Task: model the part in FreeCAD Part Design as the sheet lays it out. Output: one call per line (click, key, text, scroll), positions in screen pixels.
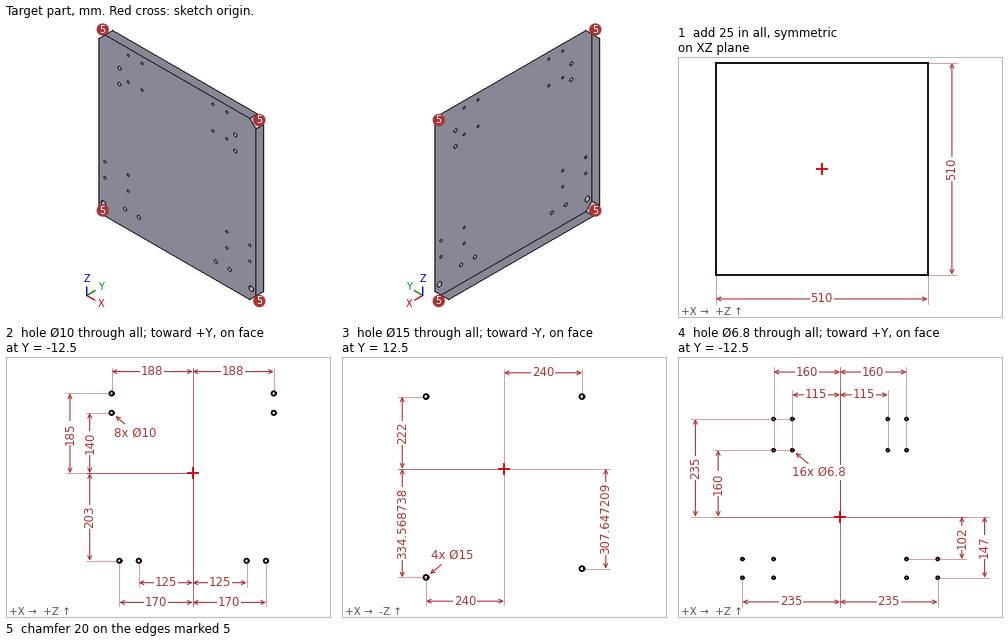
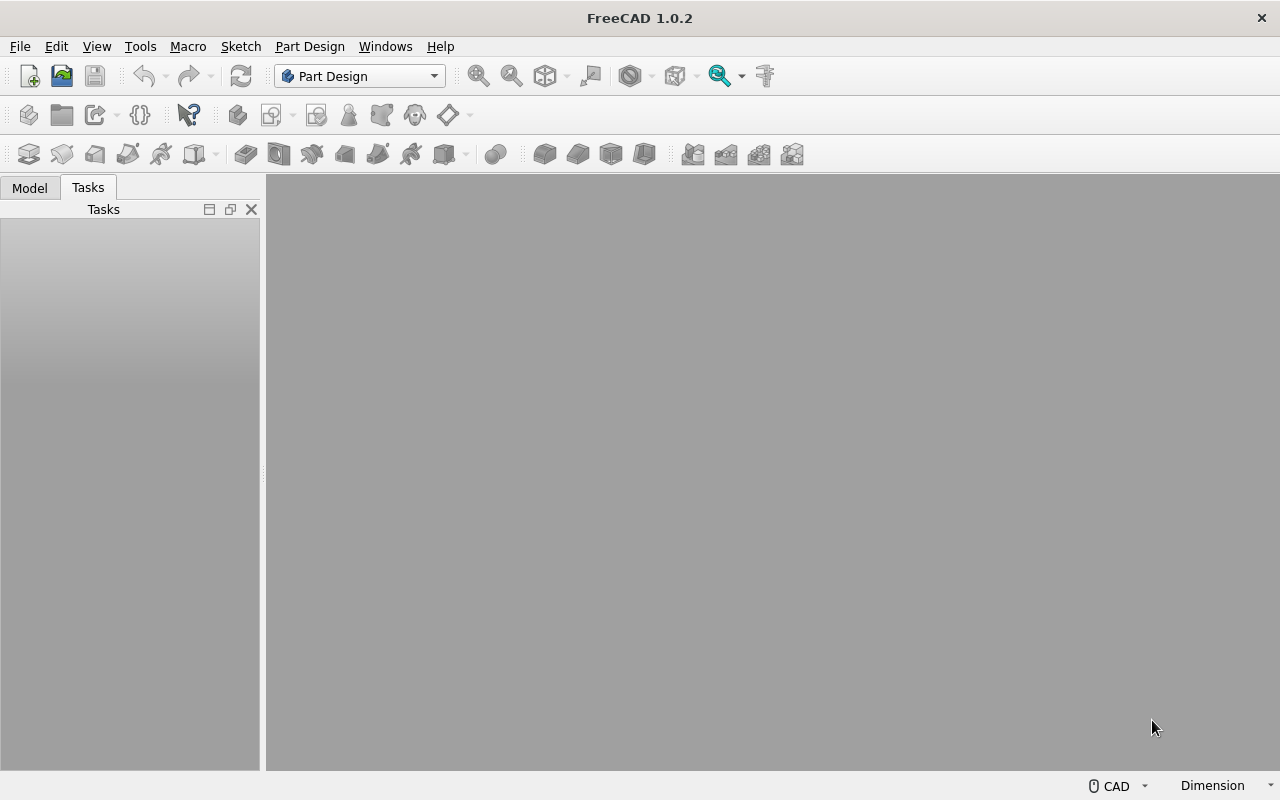
click(29, 76)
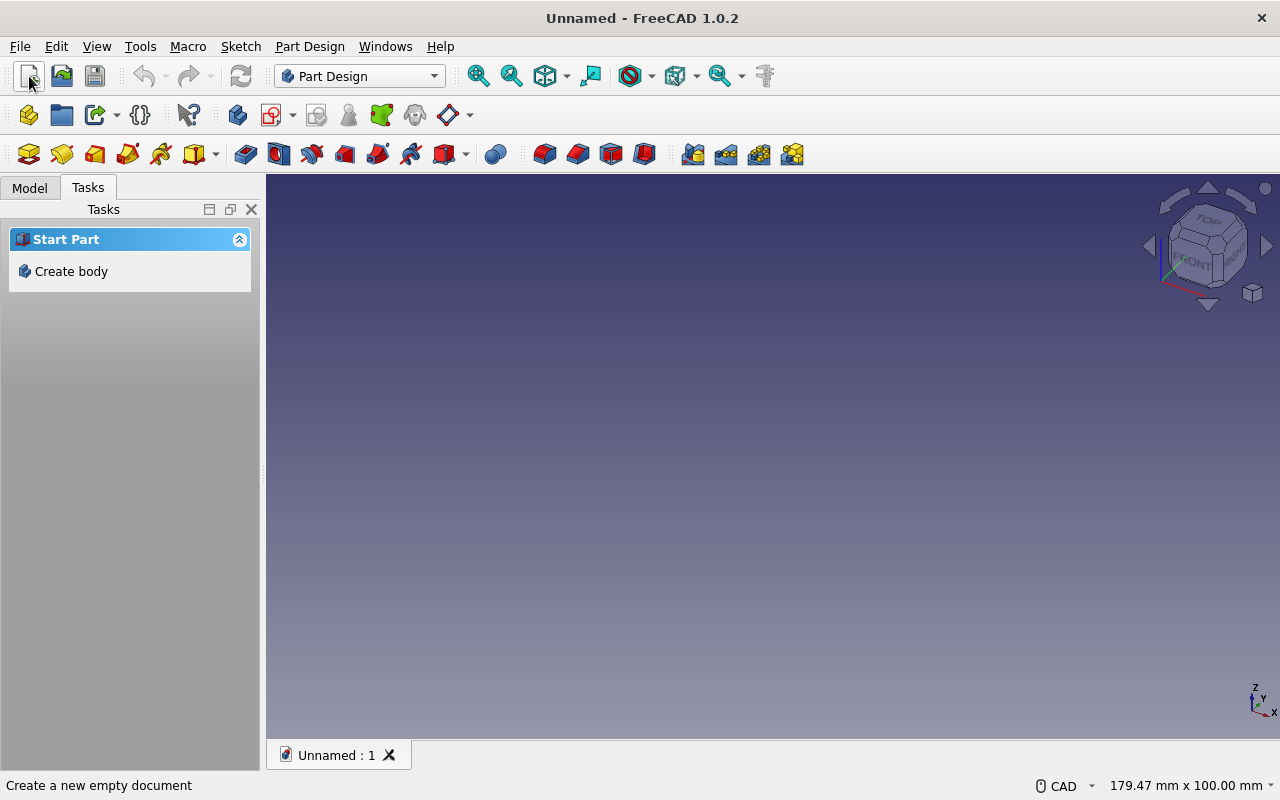
click(270, 116)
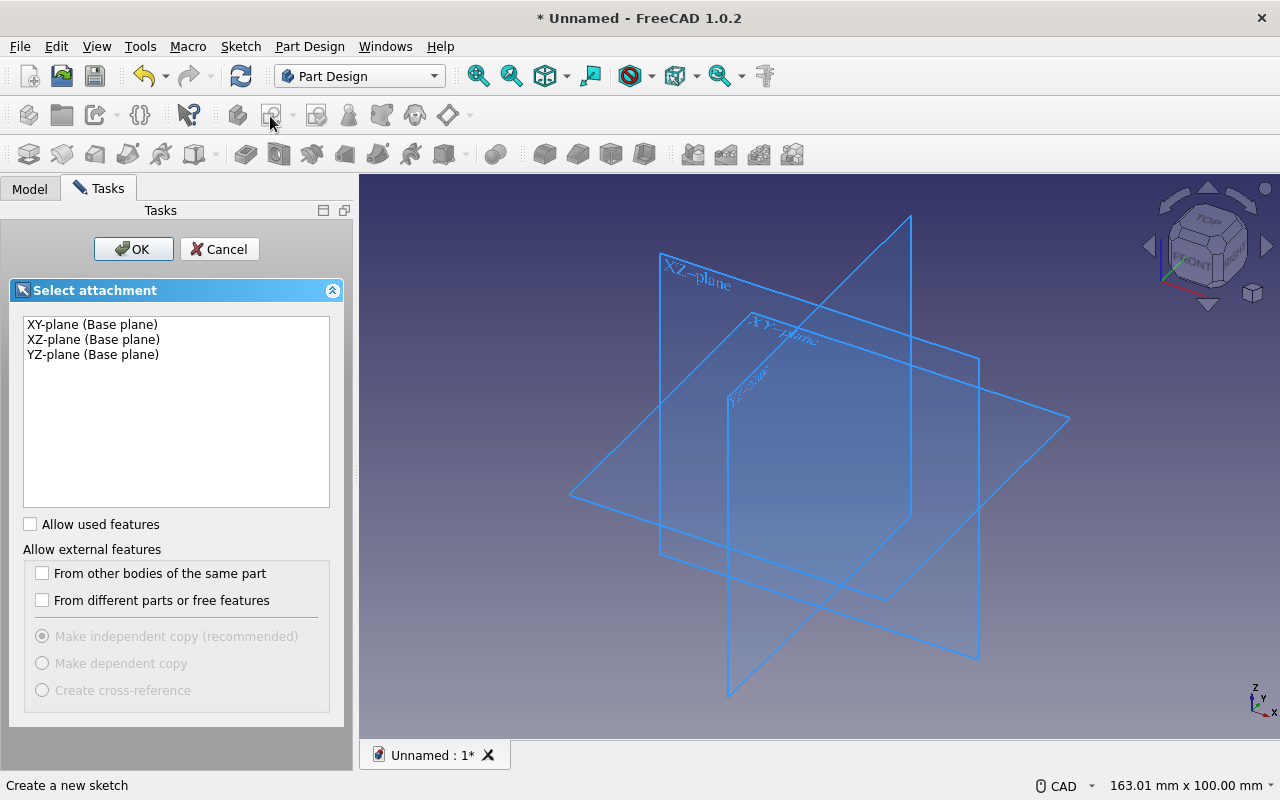
click(84, 340)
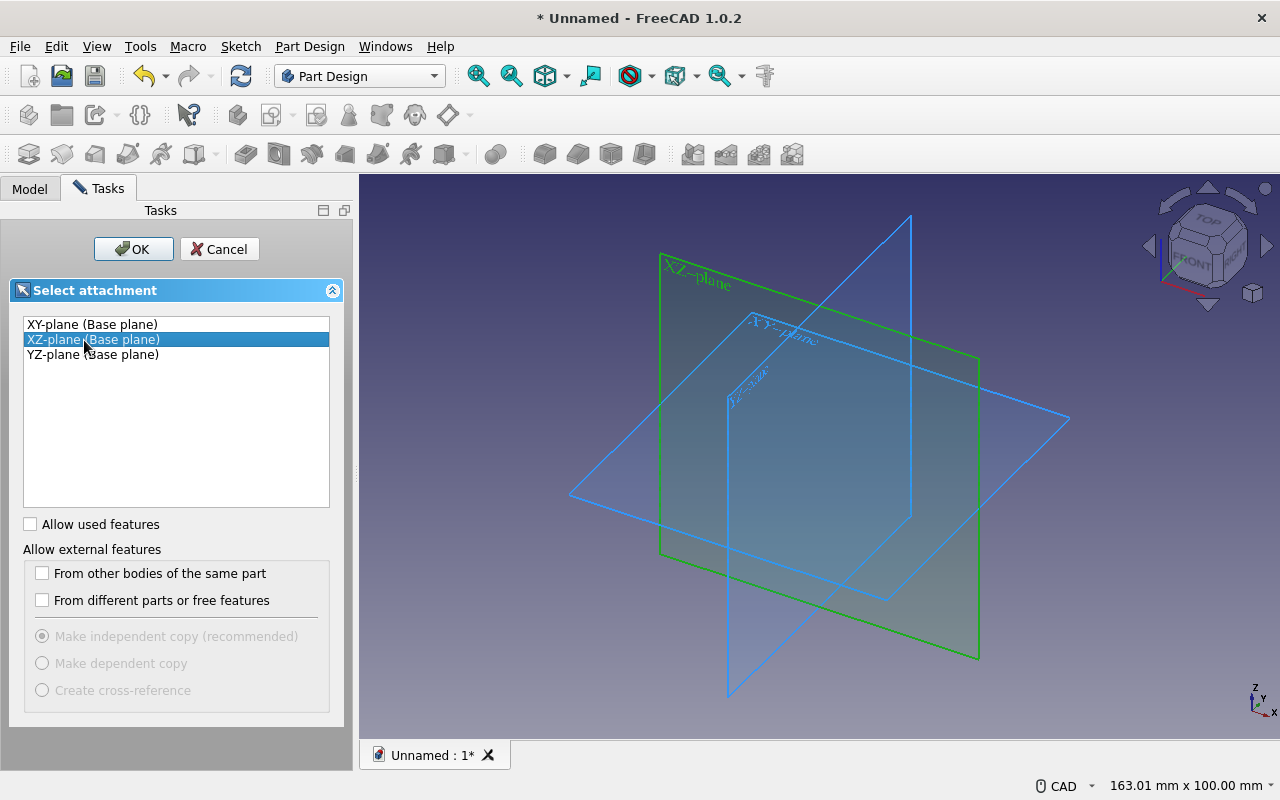
click(134, 249)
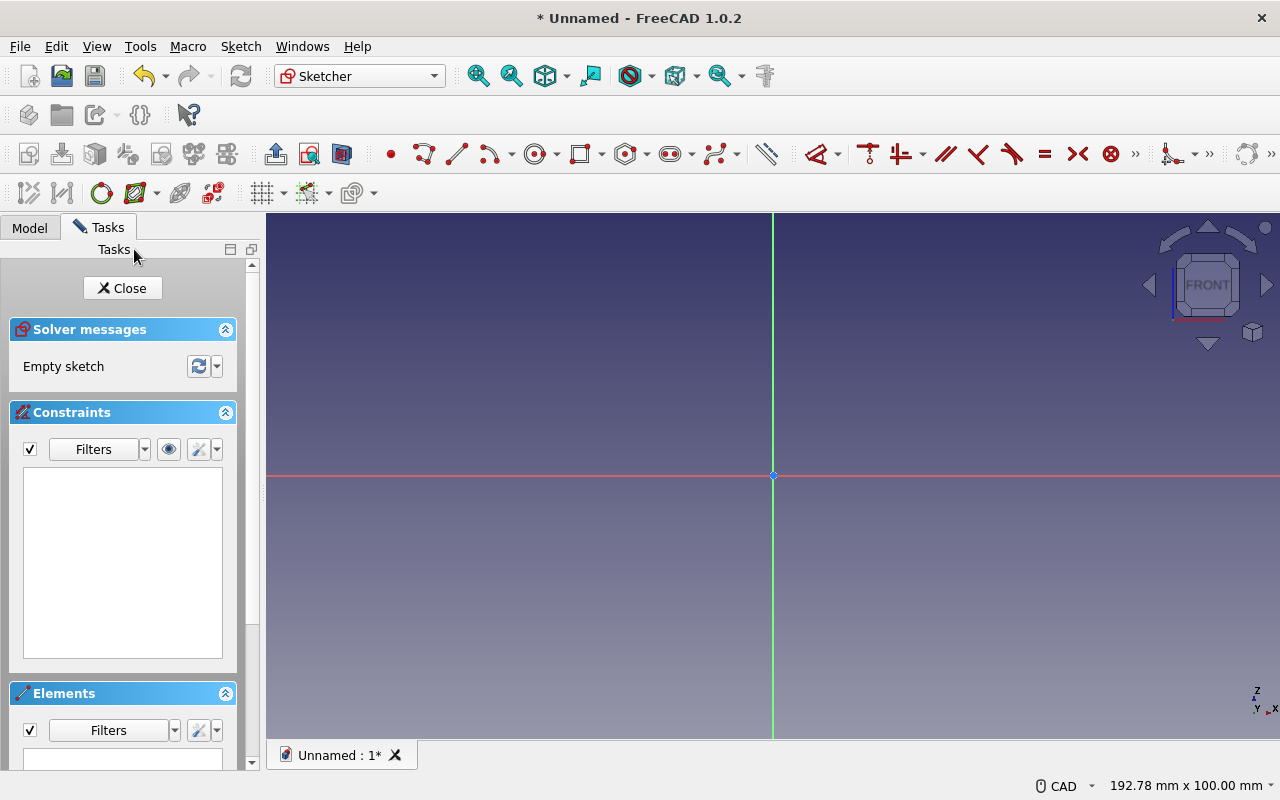
scroll(694, 476, down, 10)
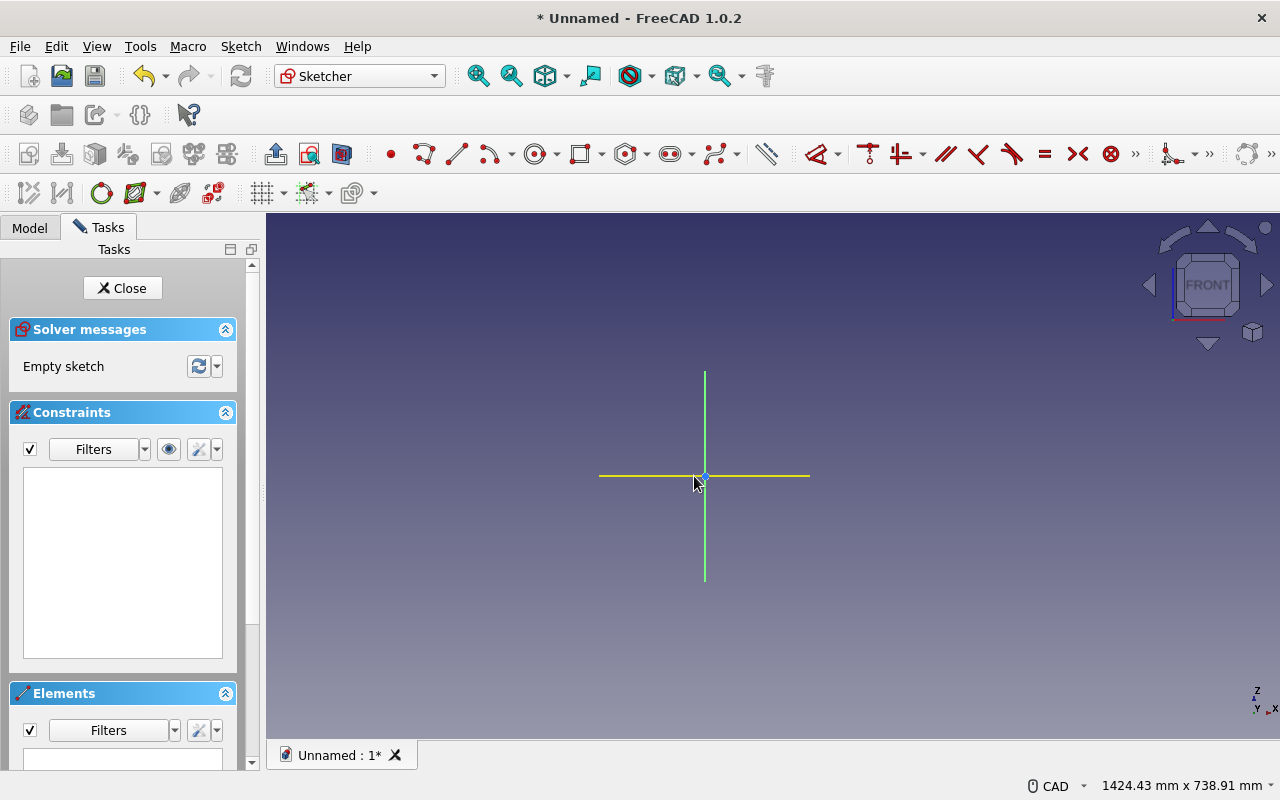
click(602, 154)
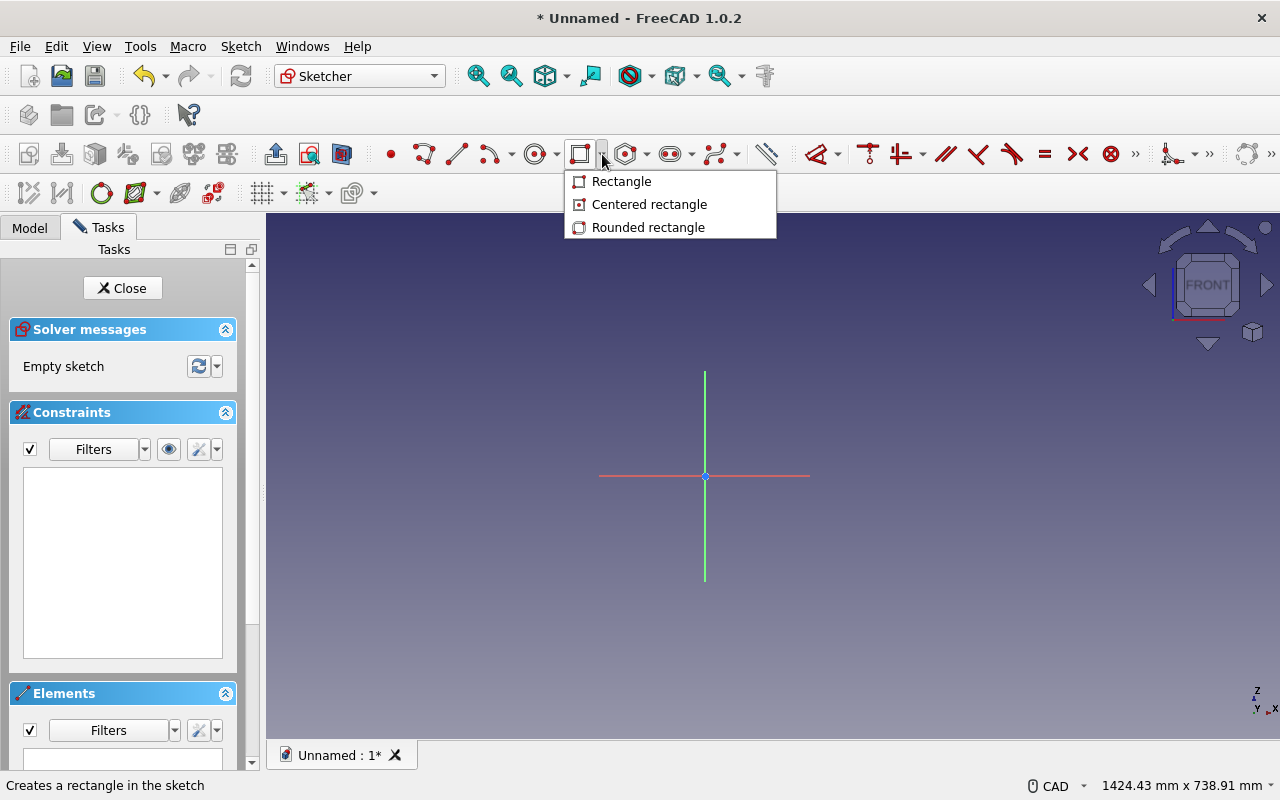
click(670, 204)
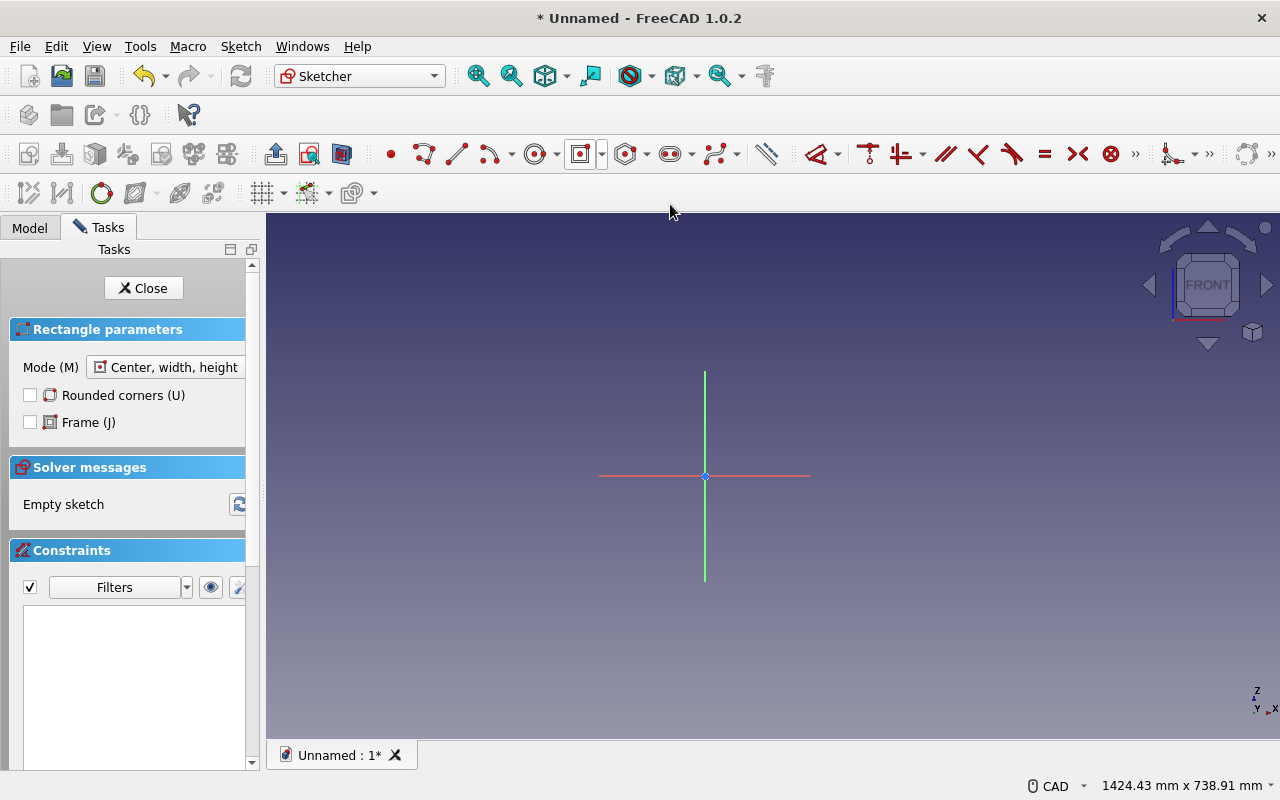
click(705, 476)
move(887, 295)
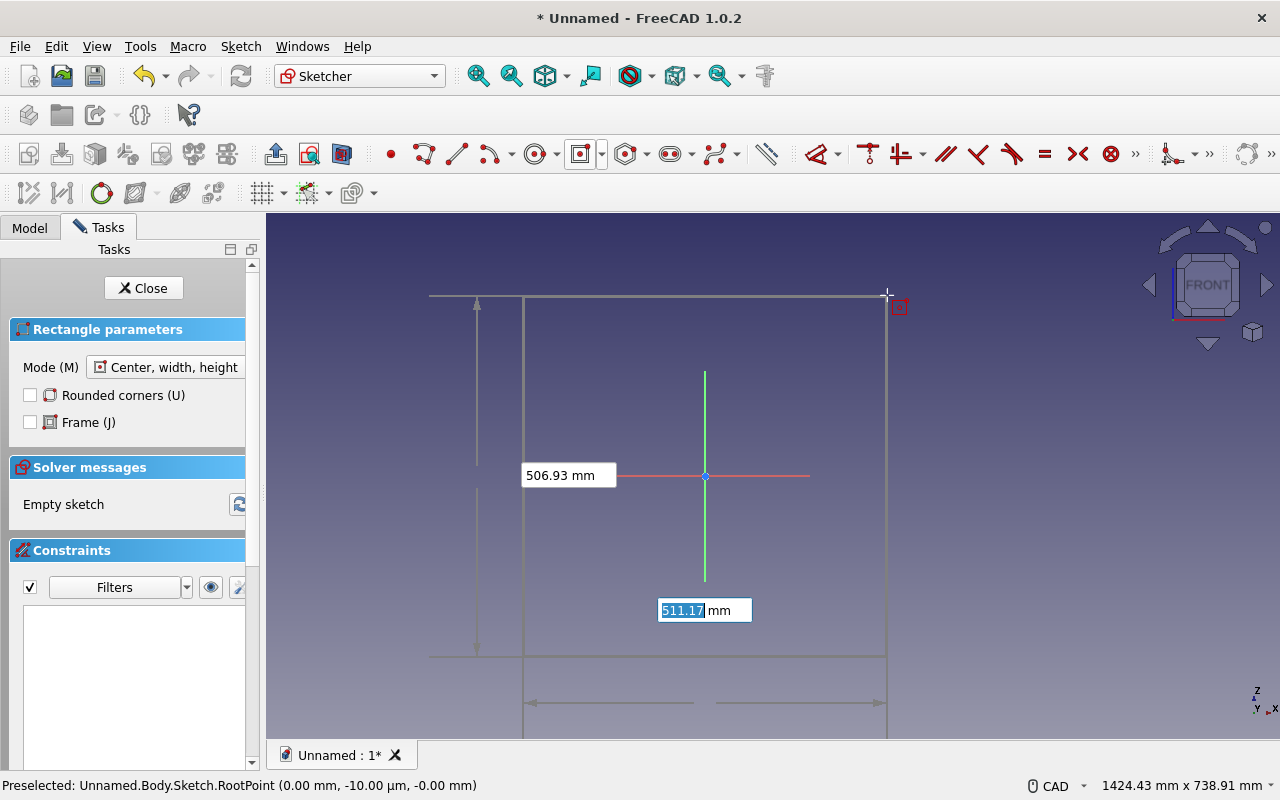
text(510)
key(Tab)
text(510)
key(Return)
key(Escape)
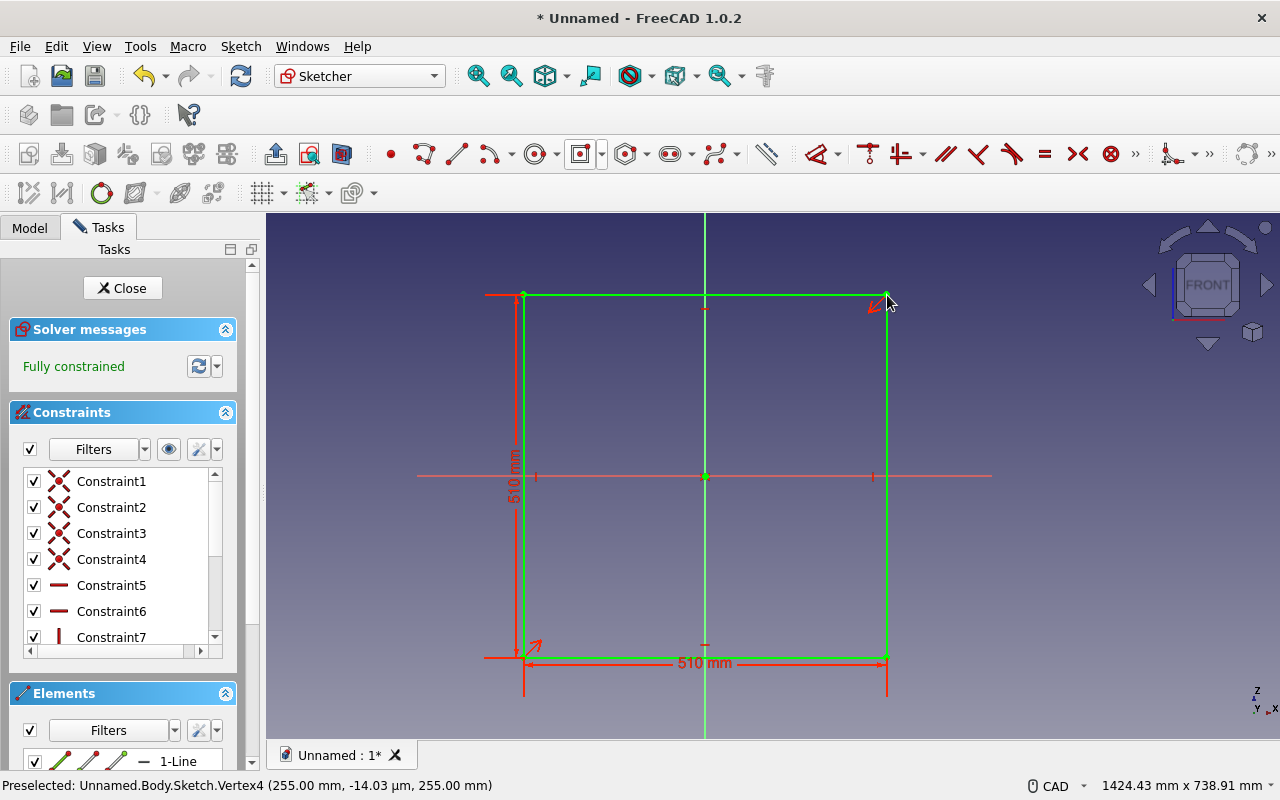
click(123, 288)